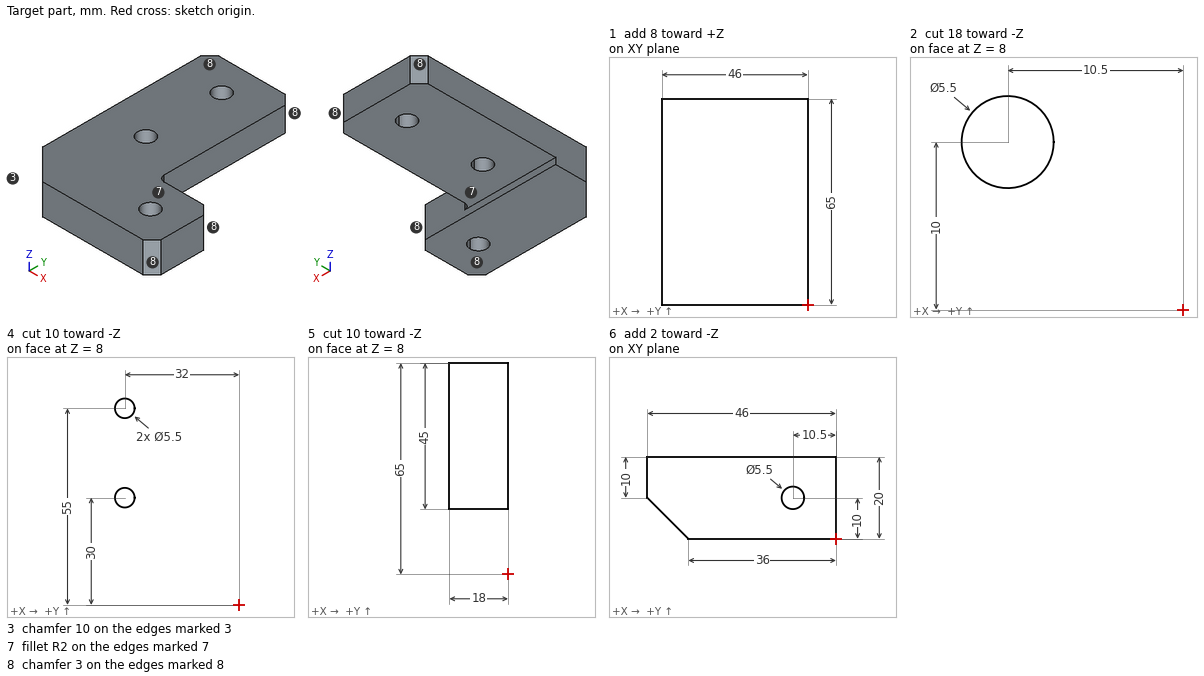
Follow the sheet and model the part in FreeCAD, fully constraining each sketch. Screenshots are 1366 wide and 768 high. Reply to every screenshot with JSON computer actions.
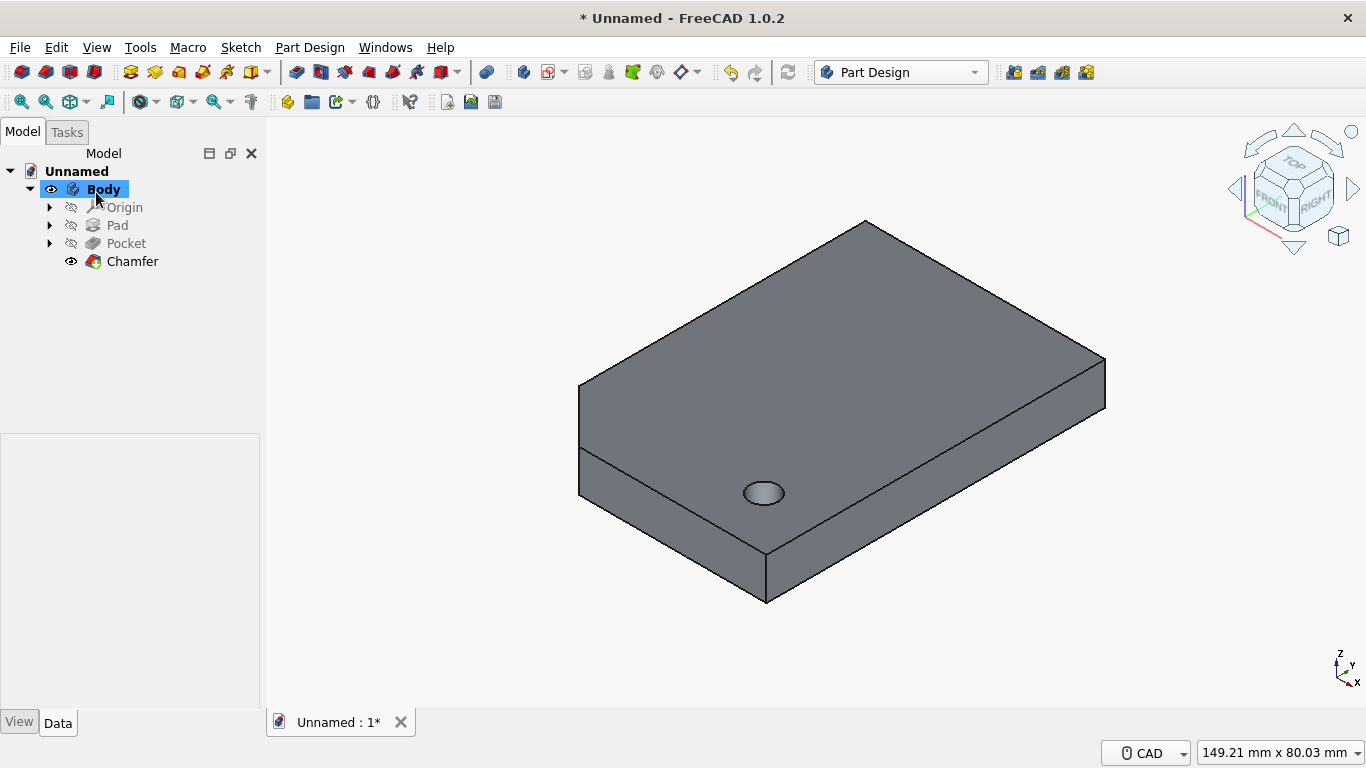
{"action": "left_click", "coordinate": [864, 359]}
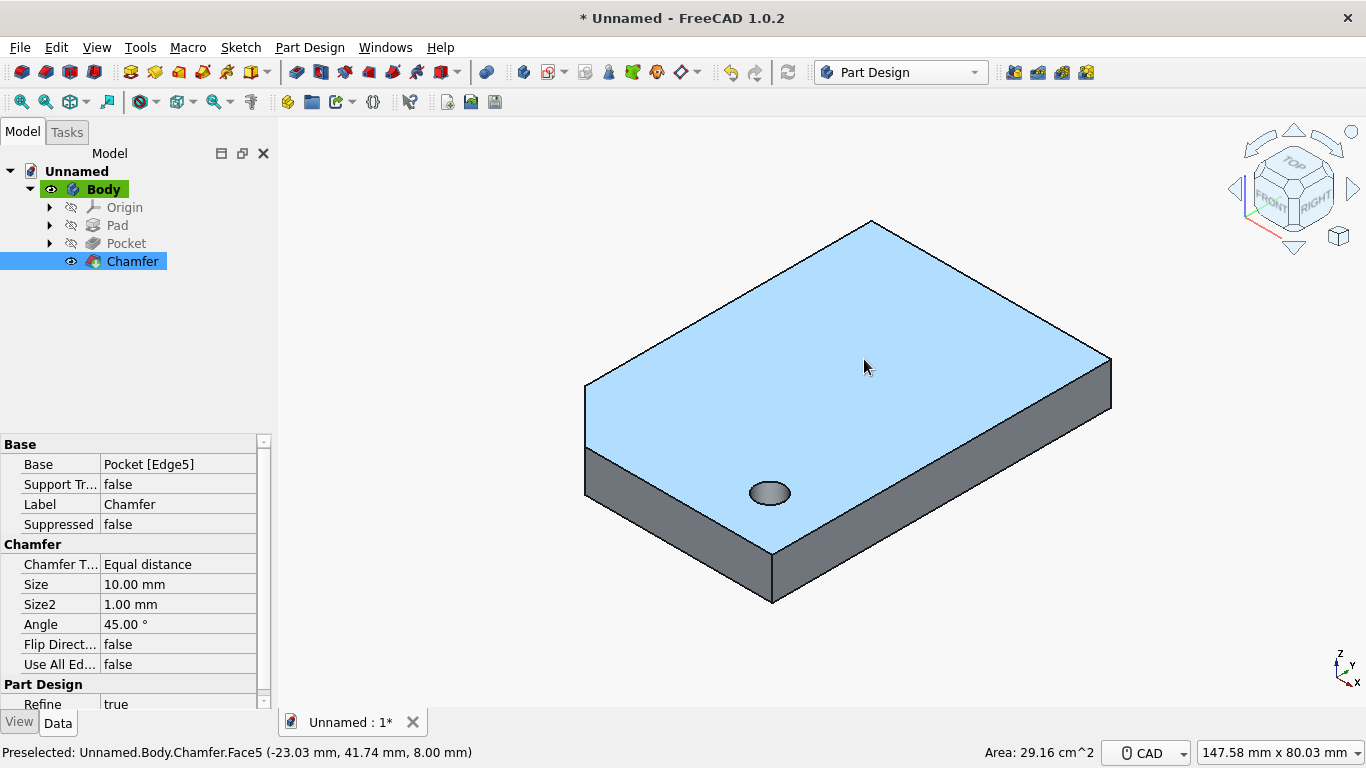
{"action": "left_click", "coordinate": [548, 72]}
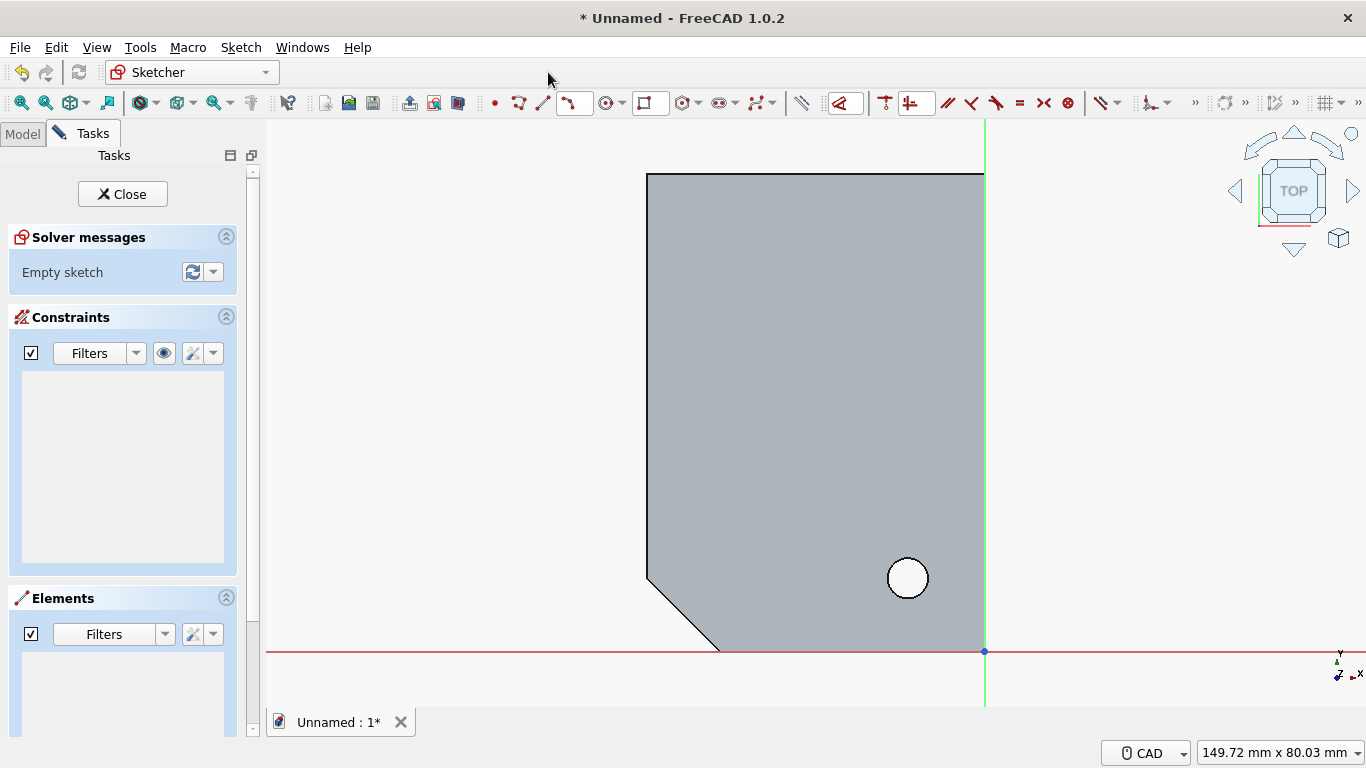
{"action": "left_click", "coordinate": [606, 104]}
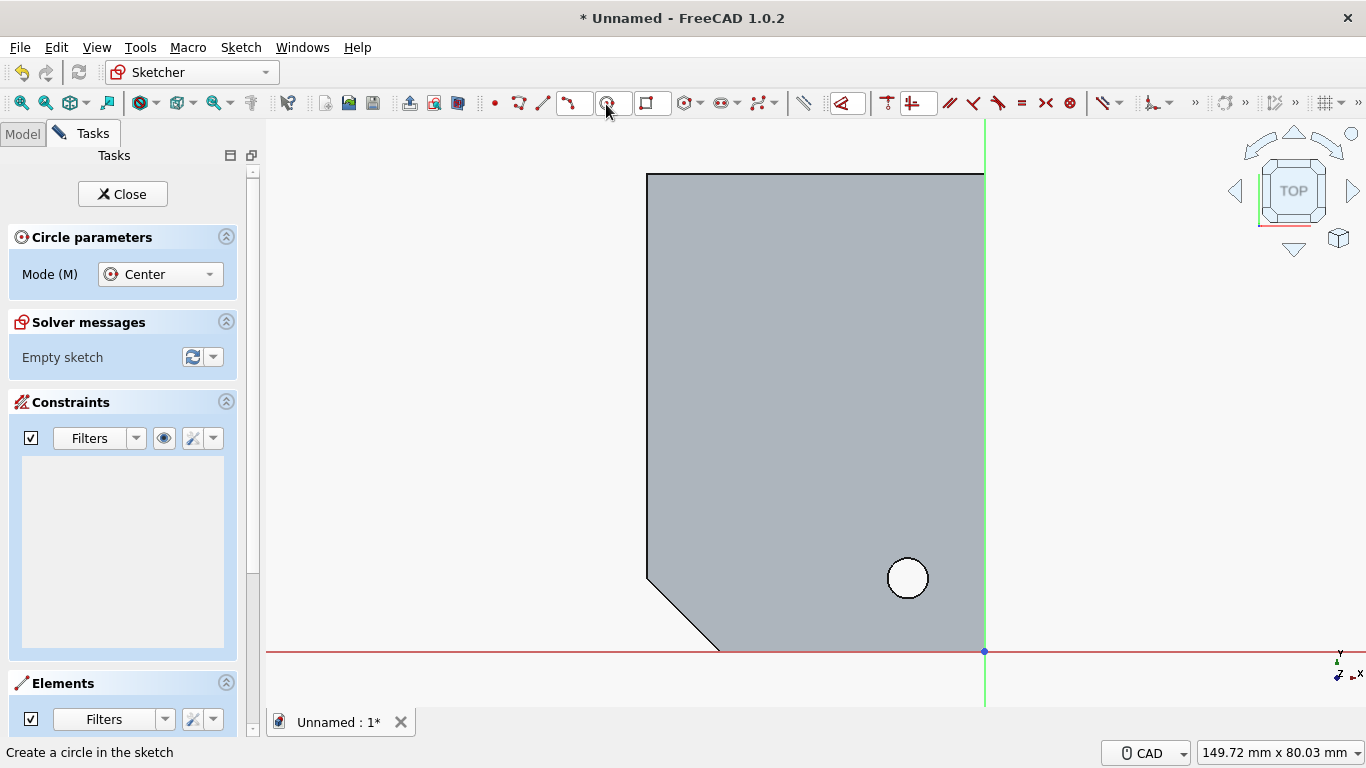
{"action": "left_click", "coordinate": [750, 248]}
{"action": "left_click", "coordinate": [764, 233]}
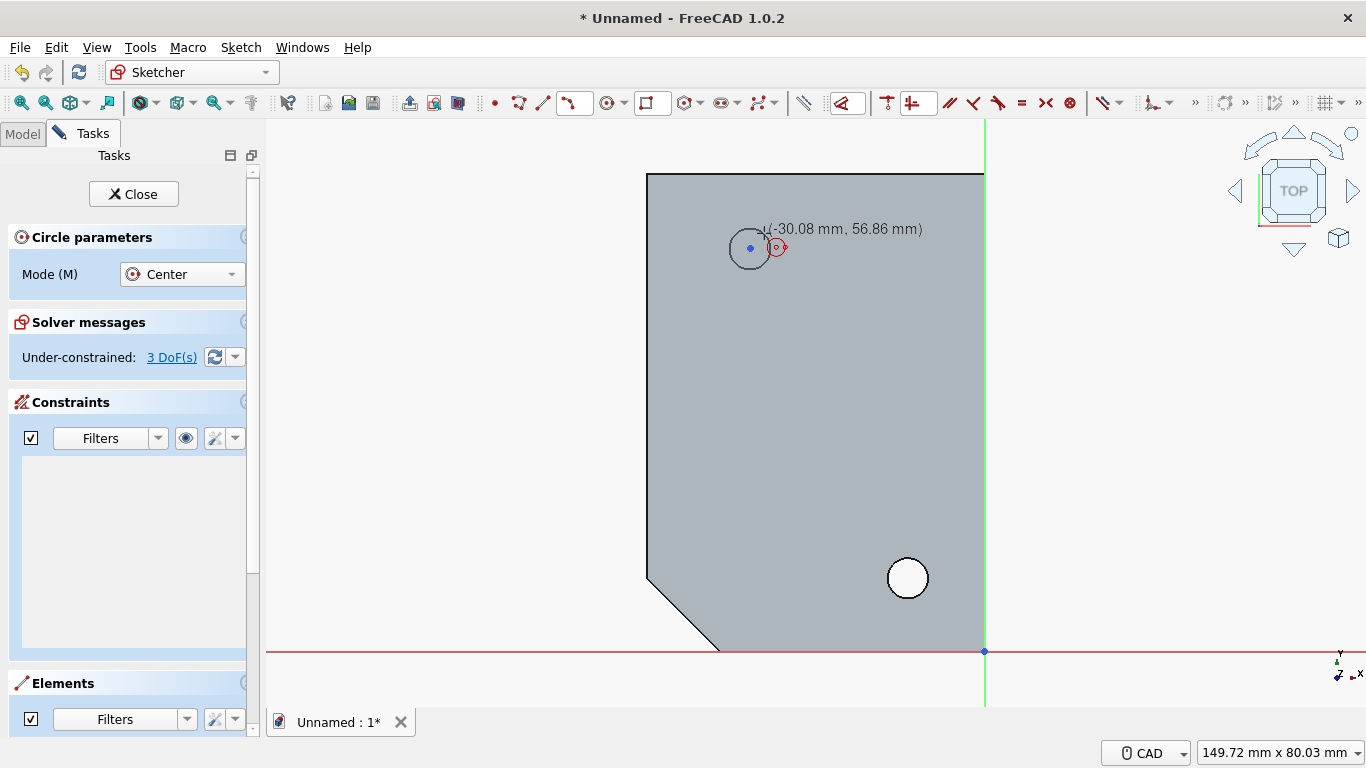
{"action": "left_click", "coordinate": [750, 431]}
{"action": "left_click", "coordinate": [764, 417]}
{"action": "key", "text": "Escape"}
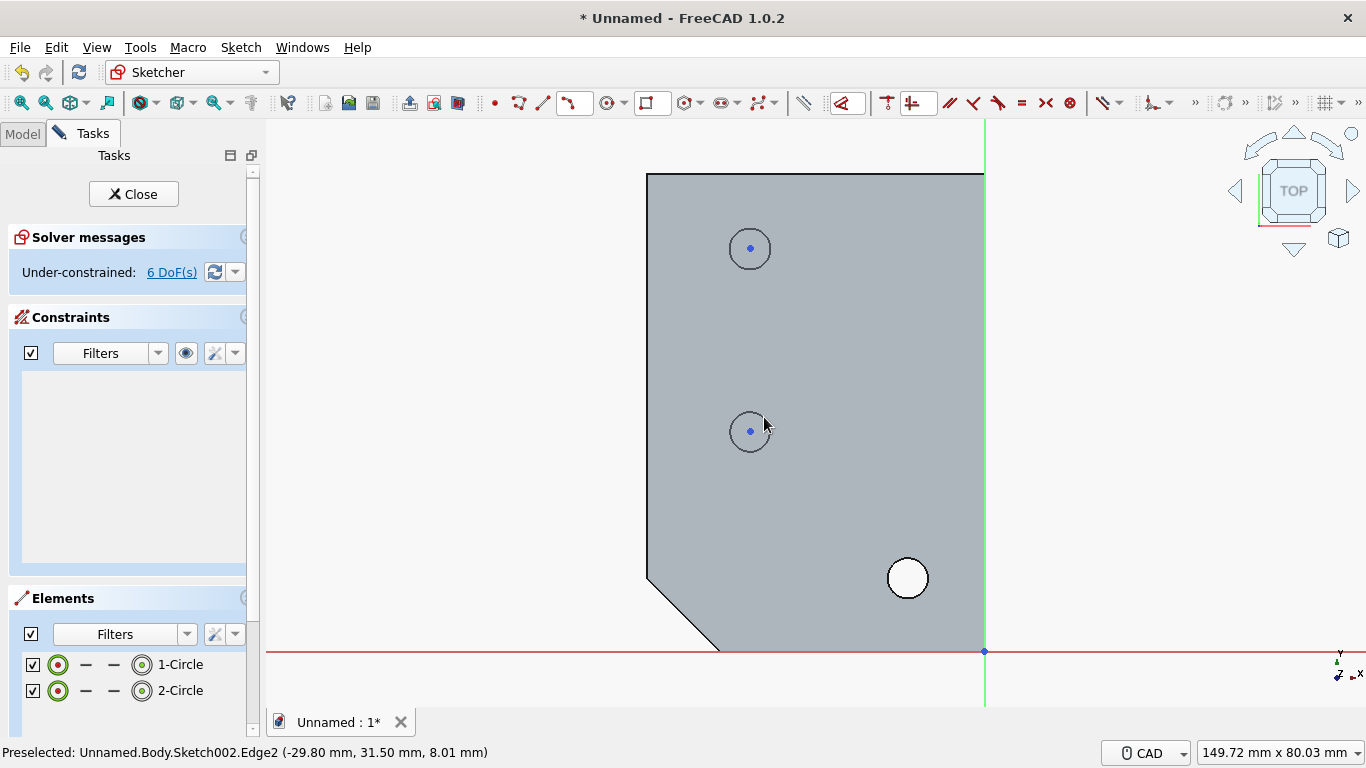
{"action": "left_click", "coordinate": [764, 234]}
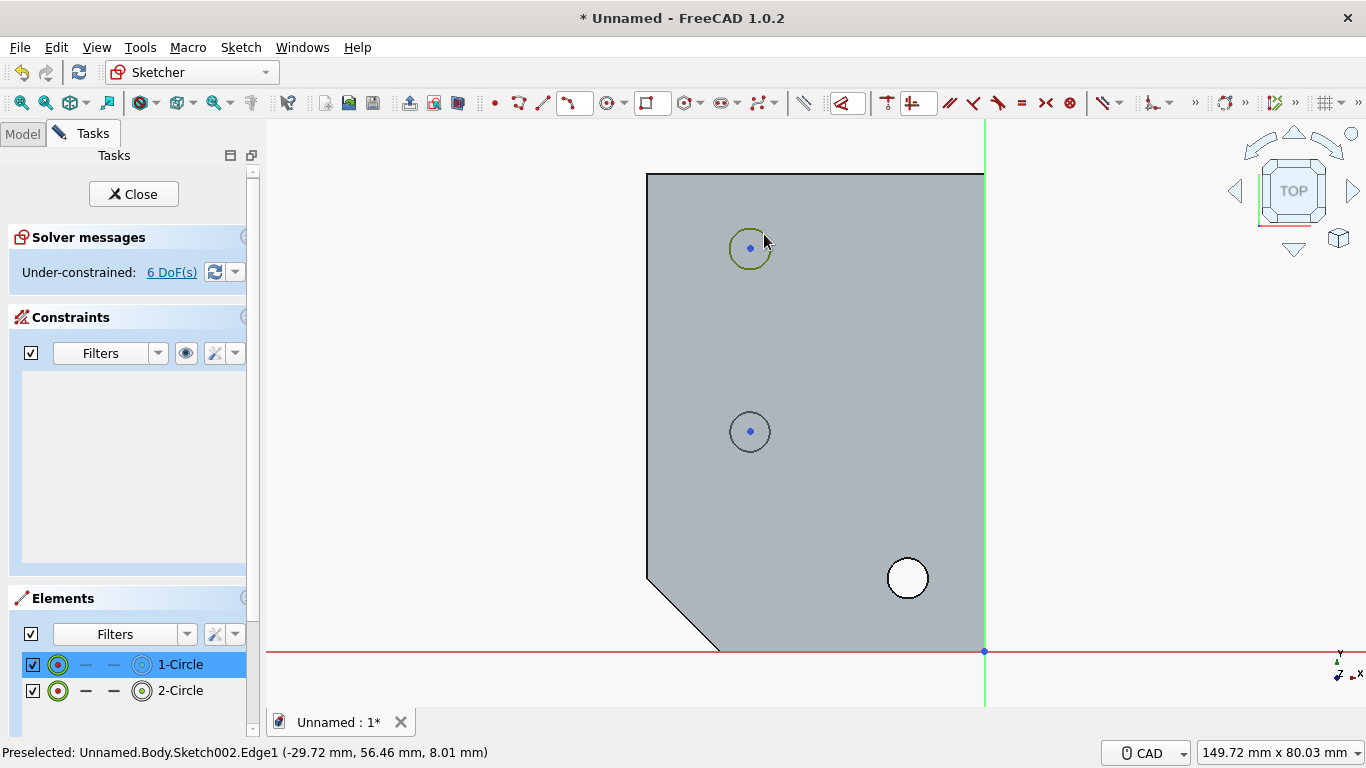
{"action": "left_click", "coordinate": [764, 418]}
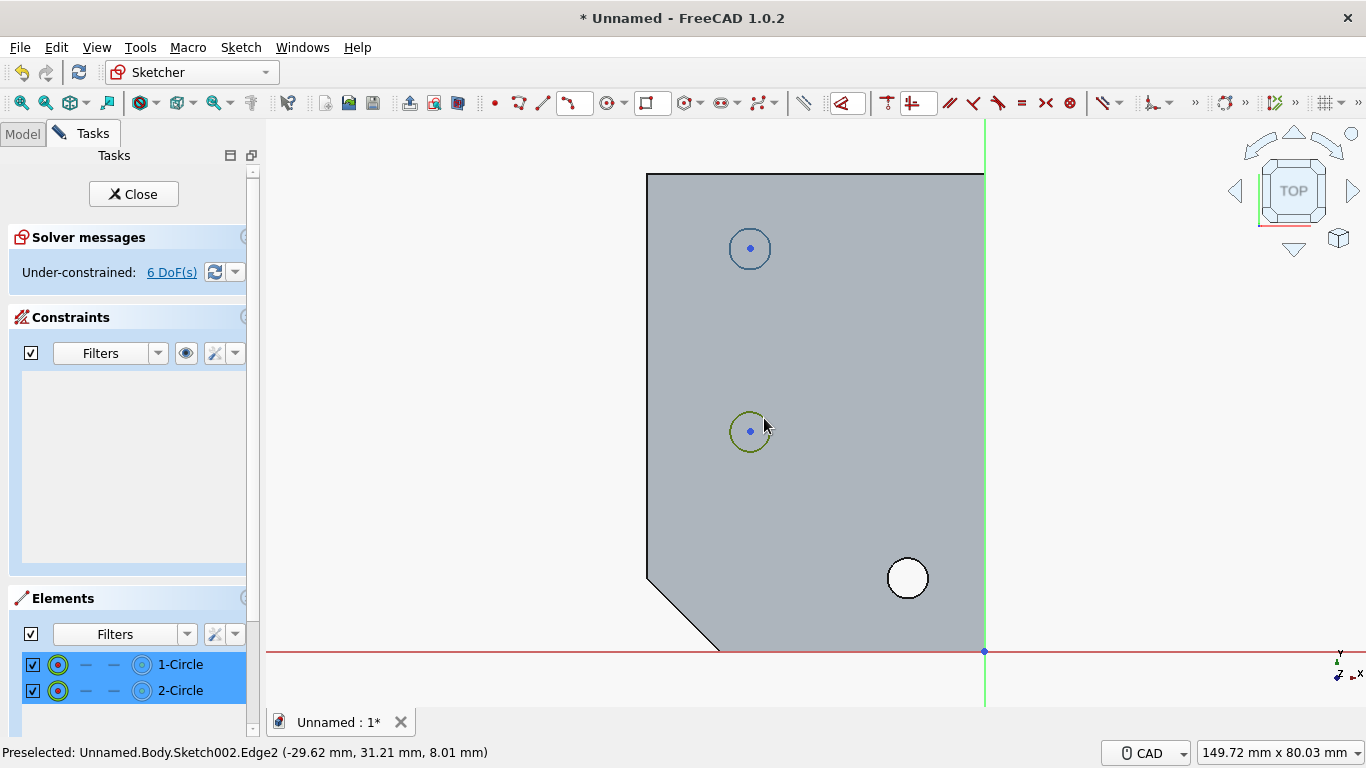
{"action": "left_click", "coordinate": [1022, 104]}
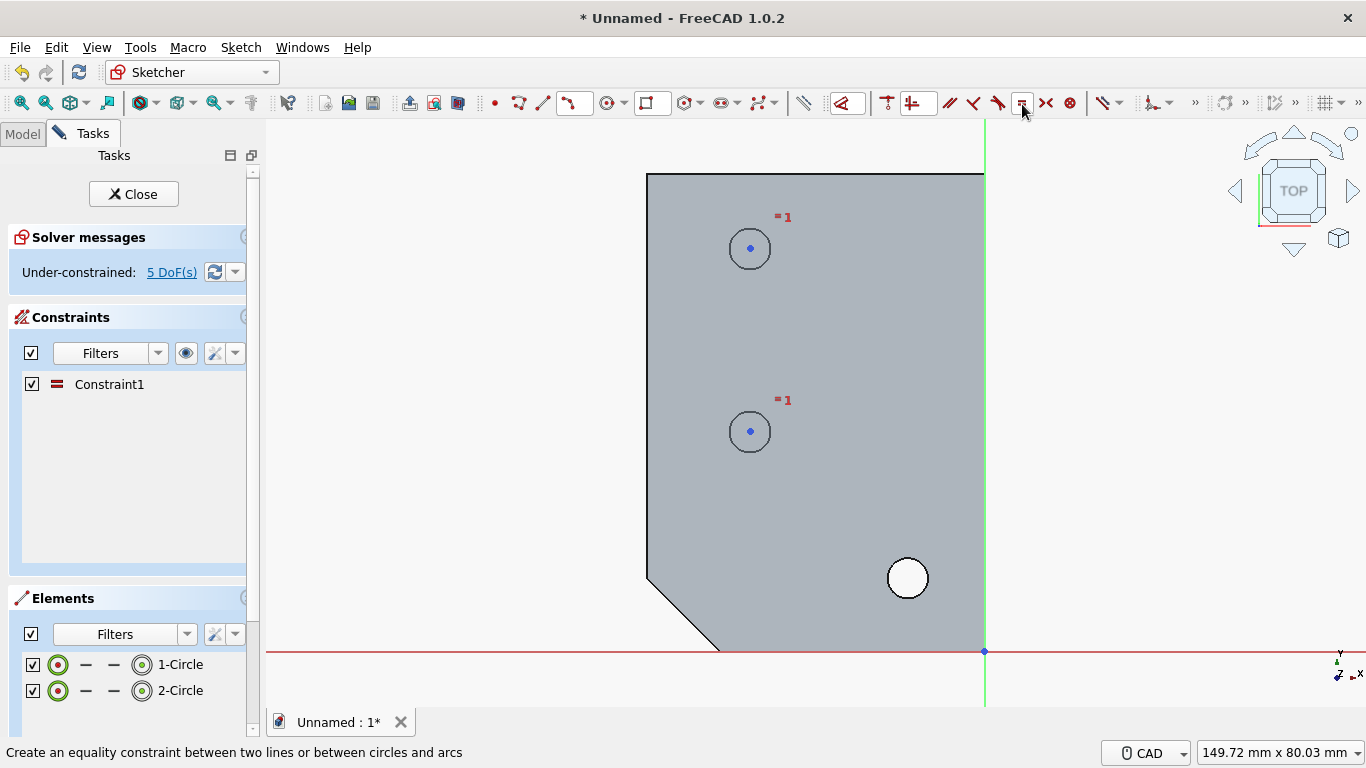
{"action": "left_click", "coordinate": [750, 249]}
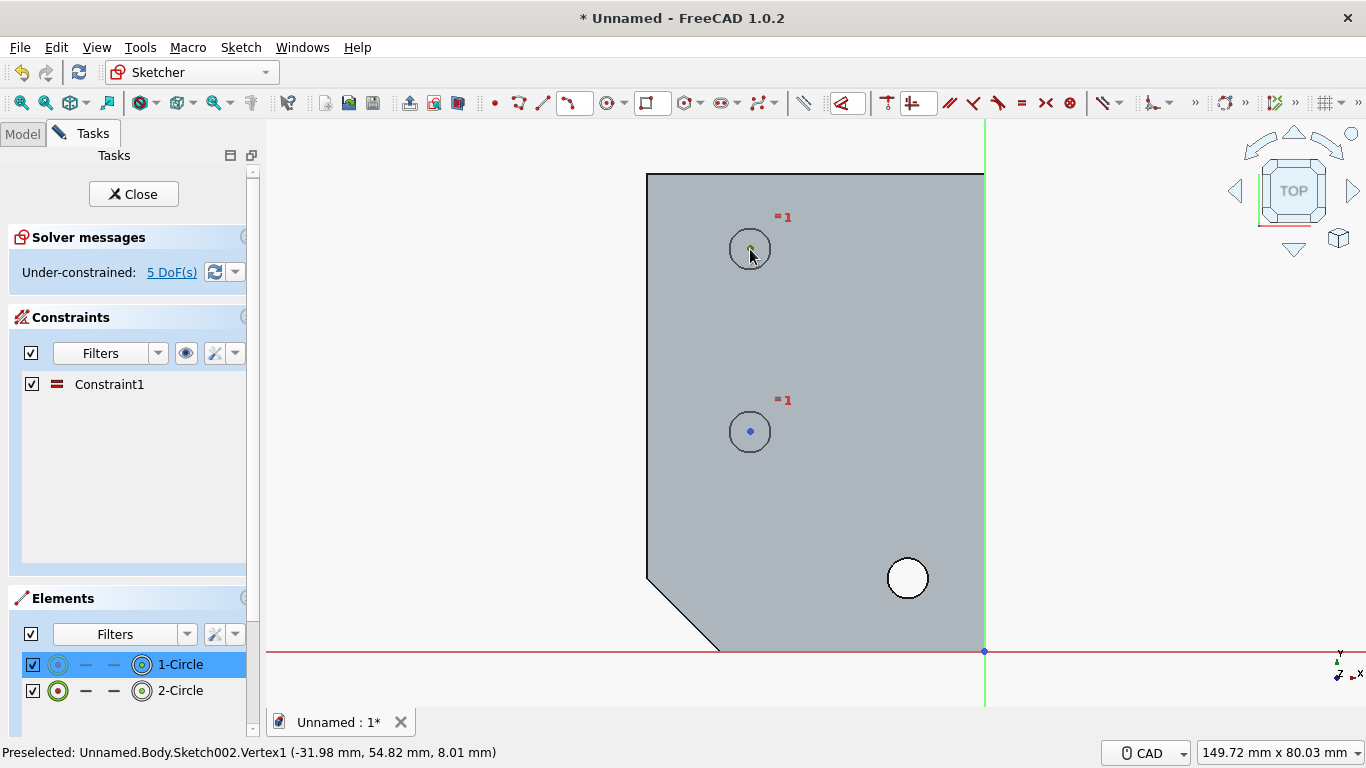
{"action": "left_click", "coordinate": [750, 432]}